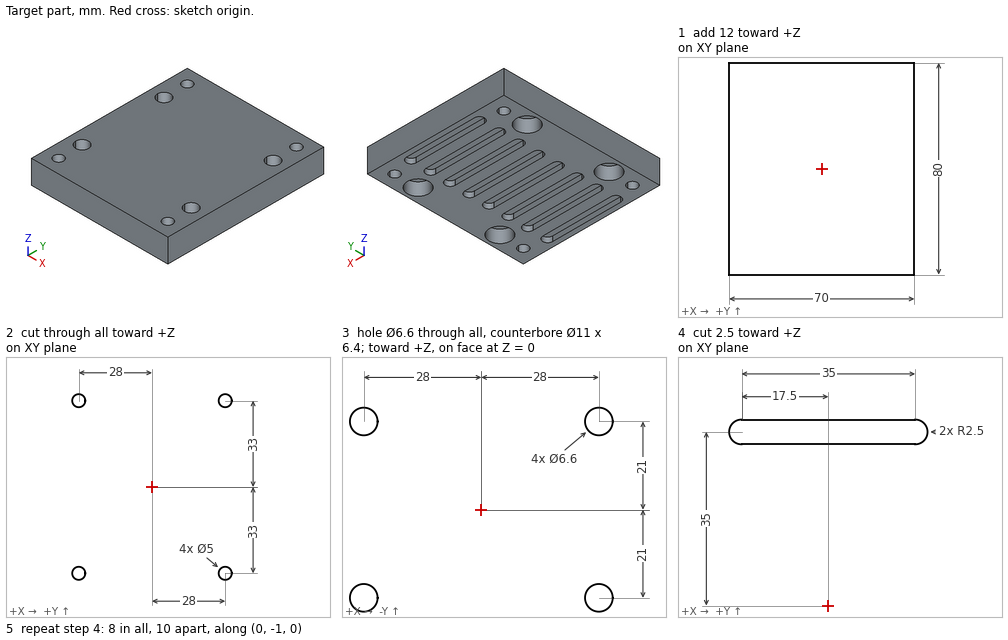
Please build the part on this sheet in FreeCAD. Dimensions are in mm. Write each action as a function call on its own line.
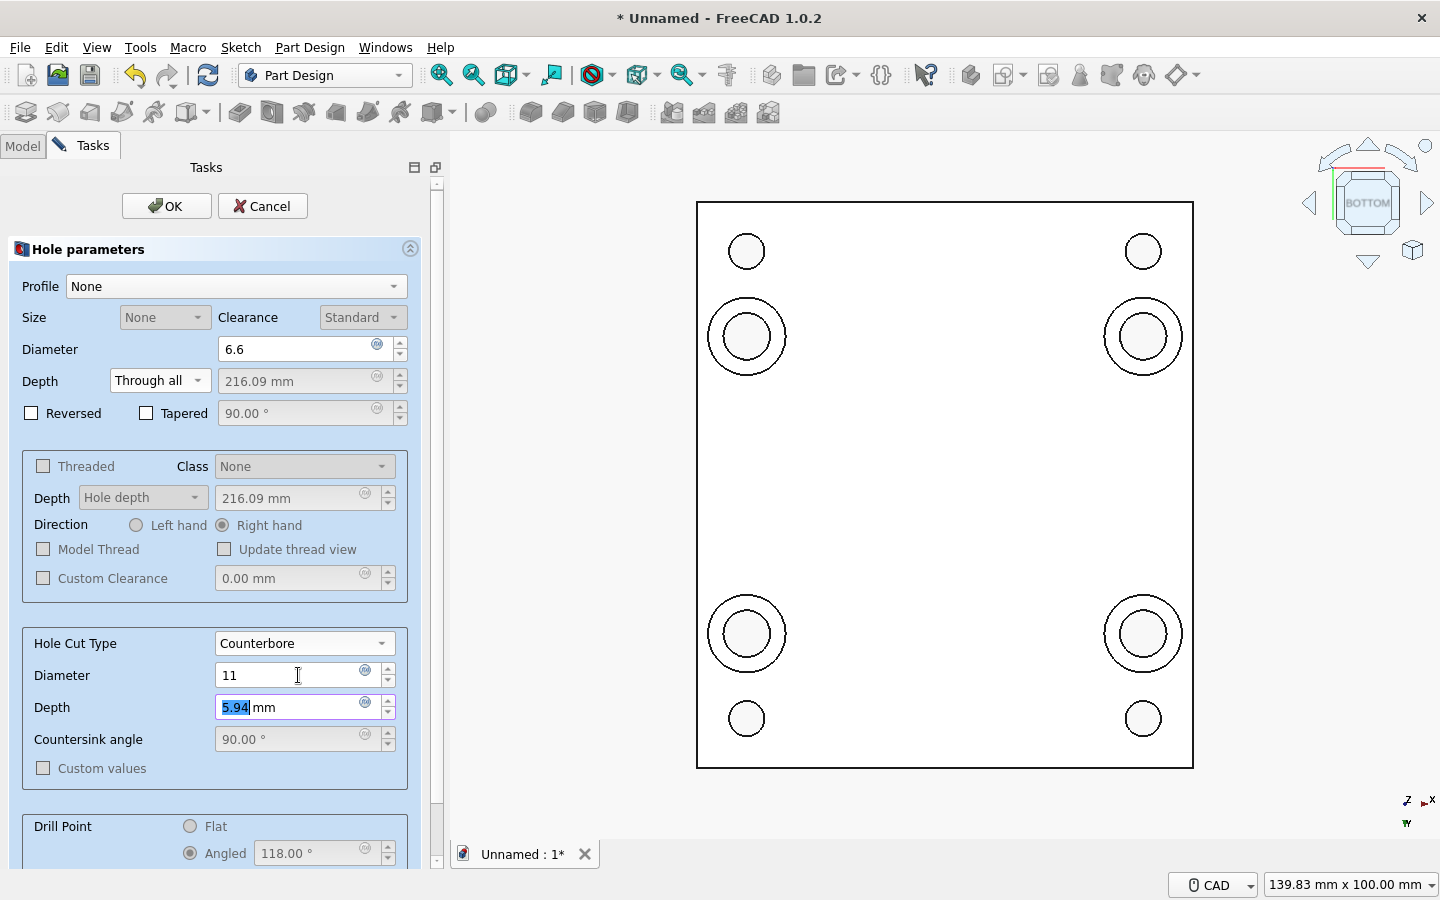
text(6.4)
key(Tab)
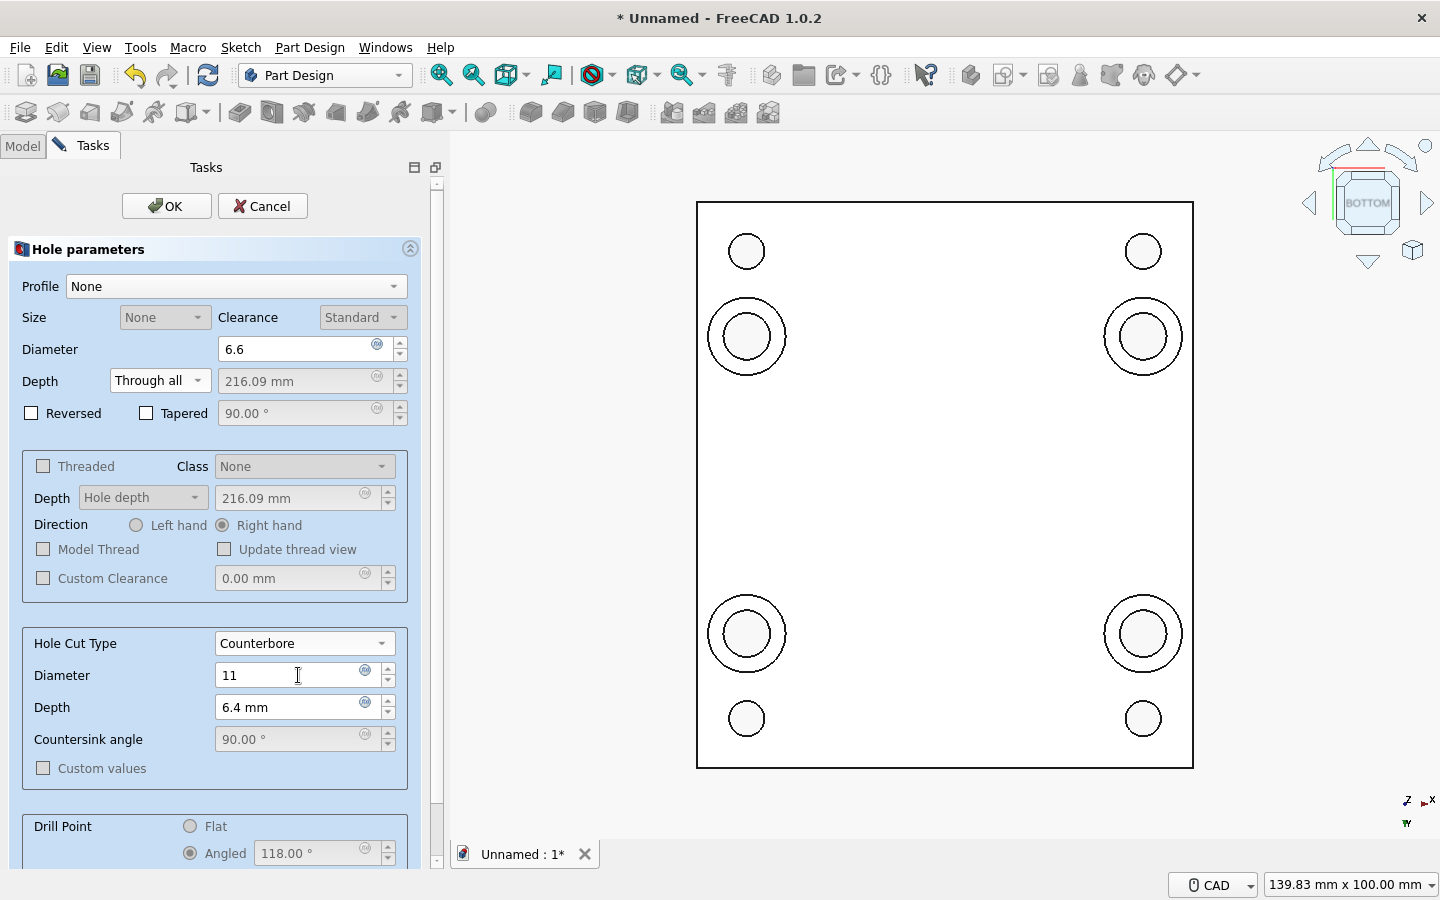
click(167, 206)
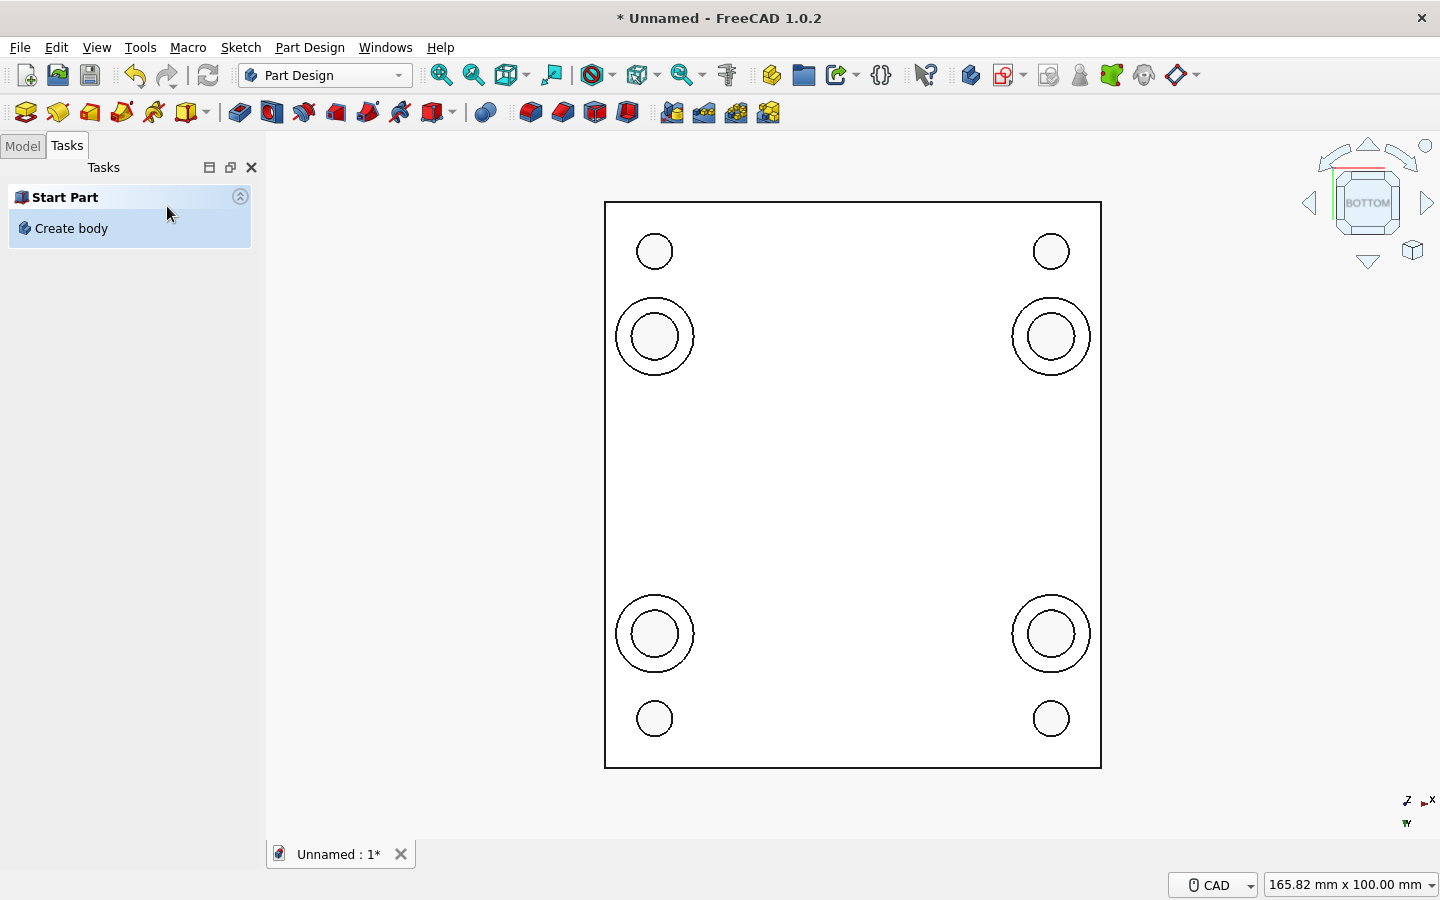
click(1004, 76)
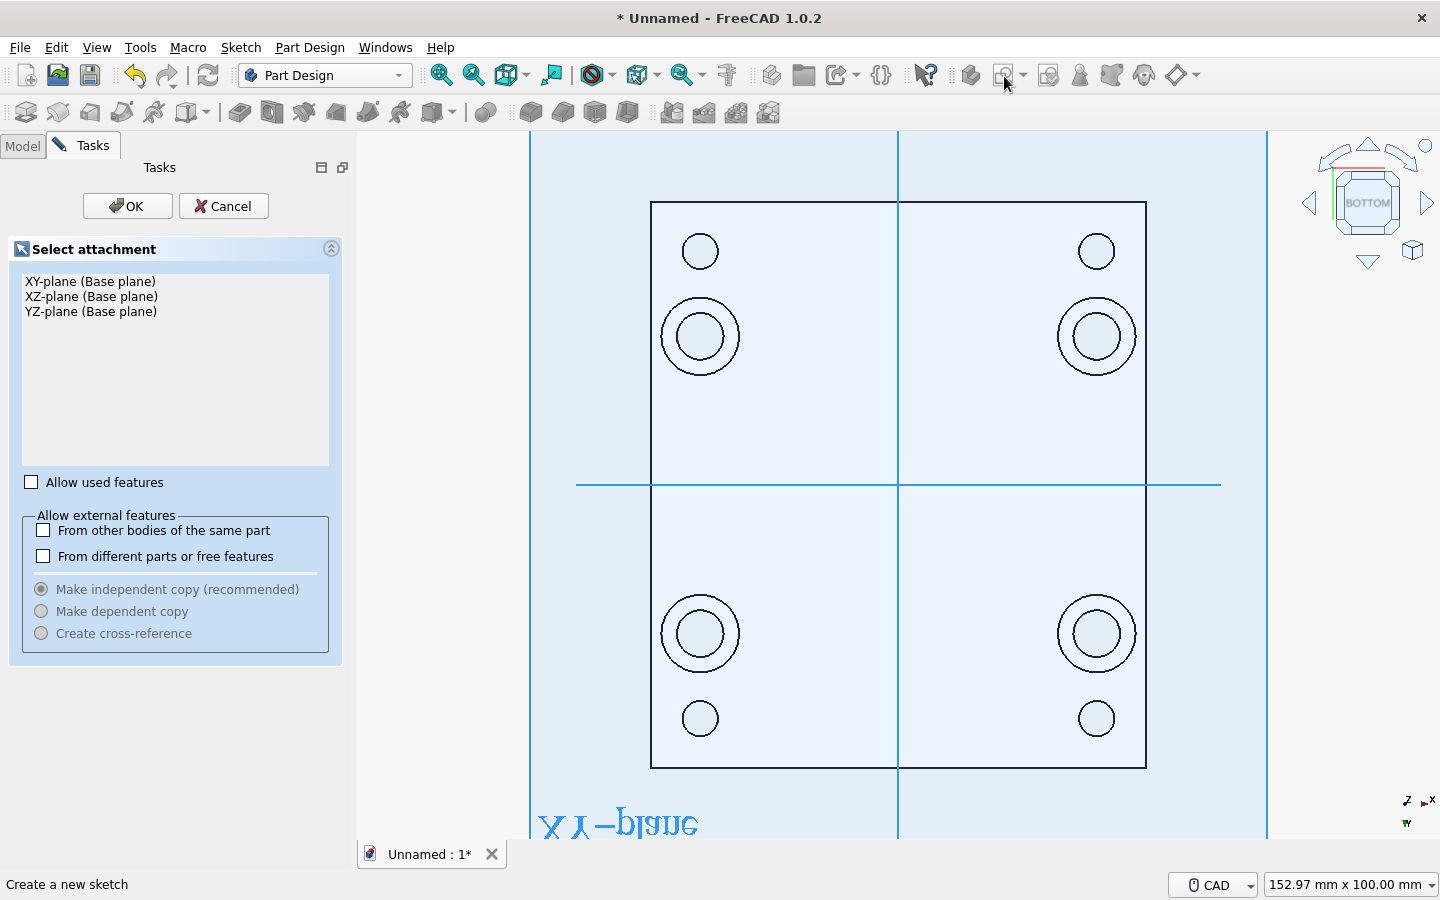
click(82, 282)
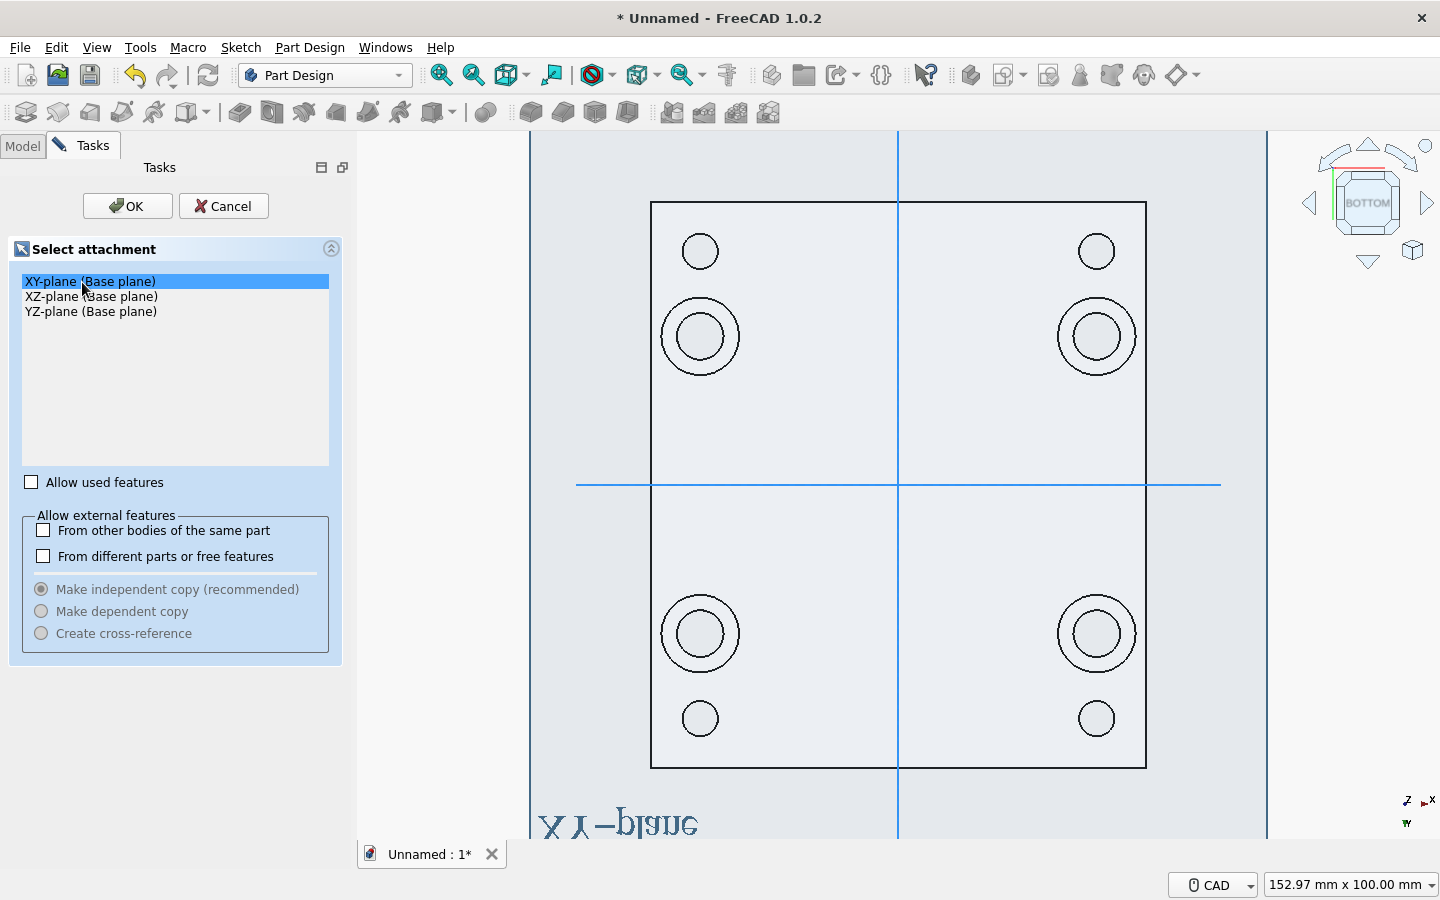
click(128, 206)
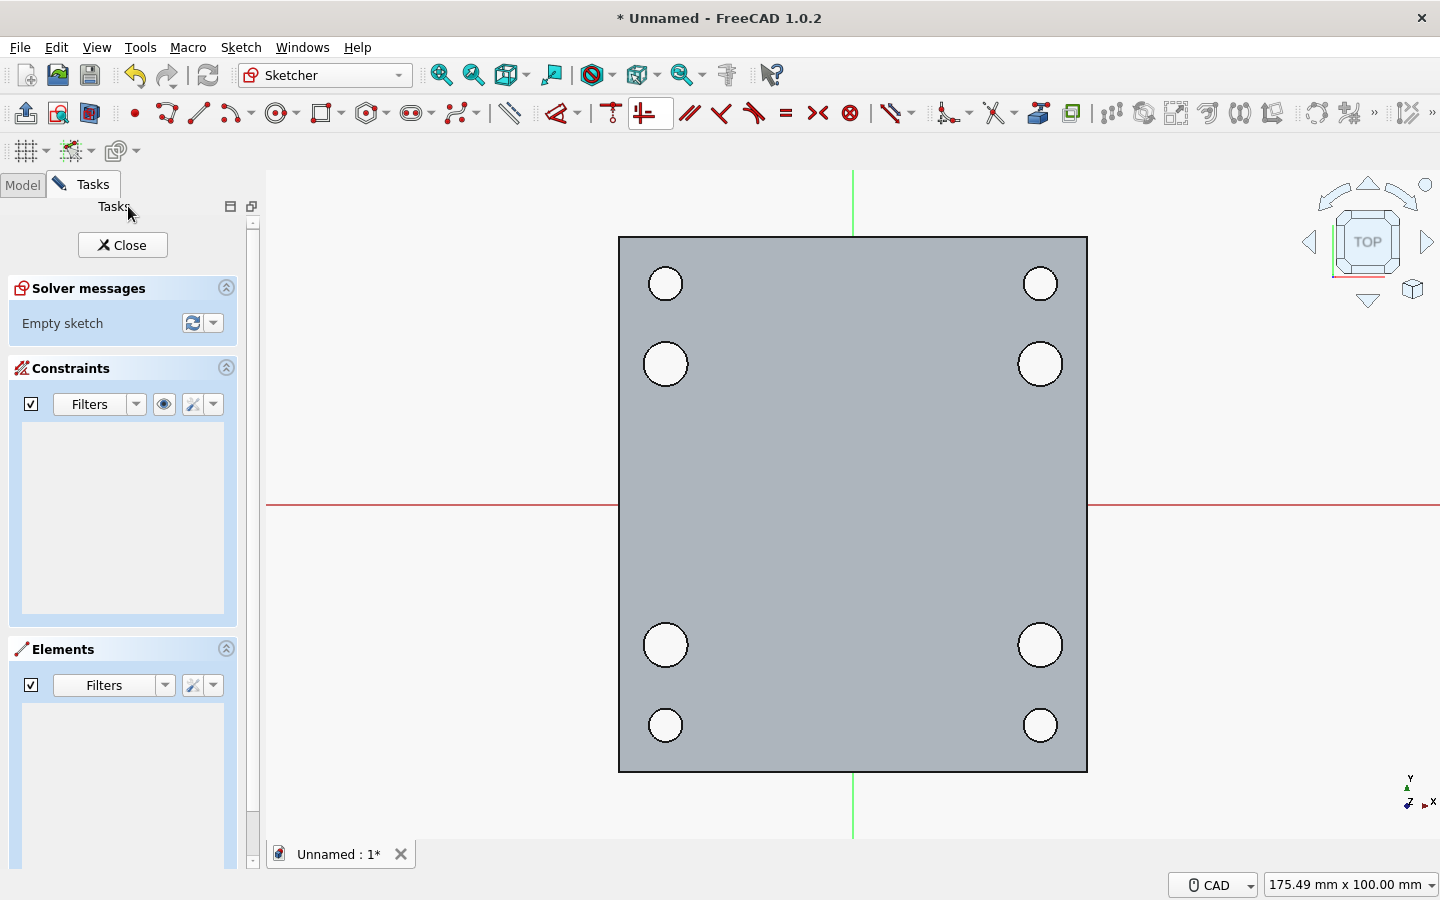
key(q)
key(s)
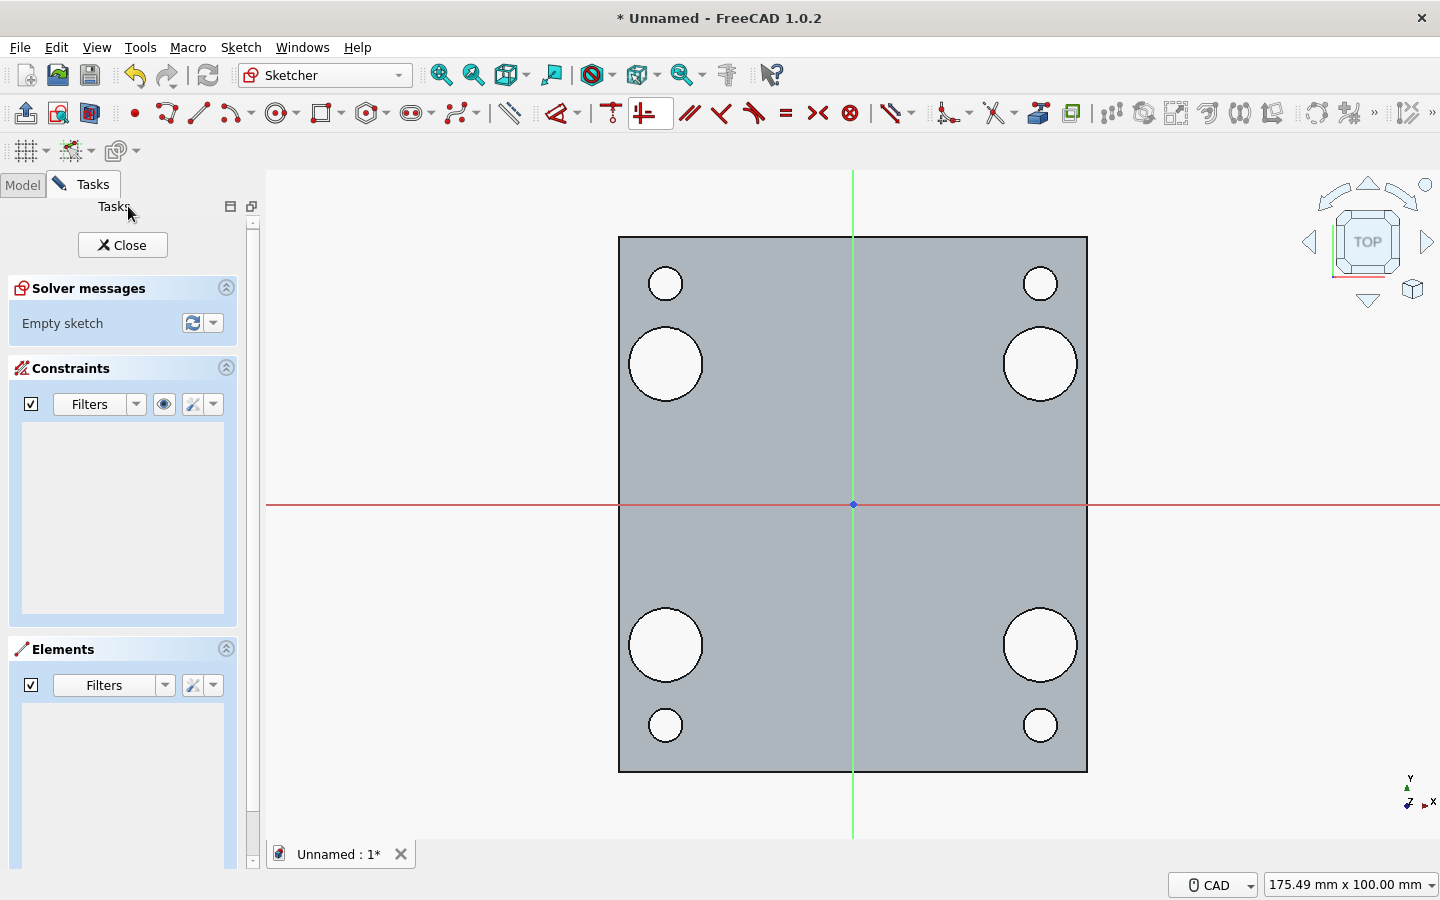
scroll(936, 226, up, 3)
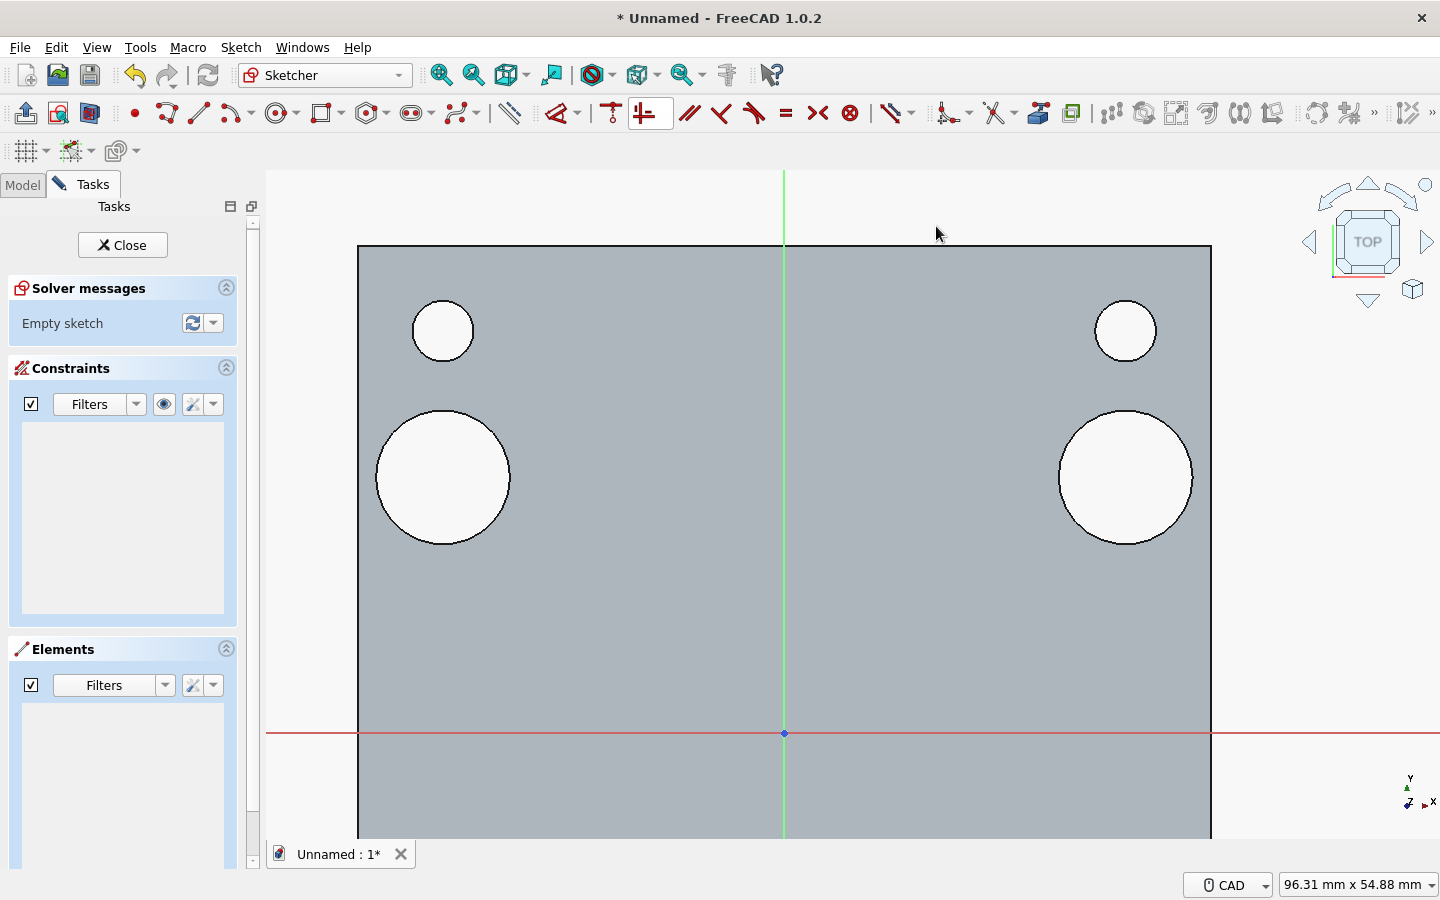
click(412, 114)